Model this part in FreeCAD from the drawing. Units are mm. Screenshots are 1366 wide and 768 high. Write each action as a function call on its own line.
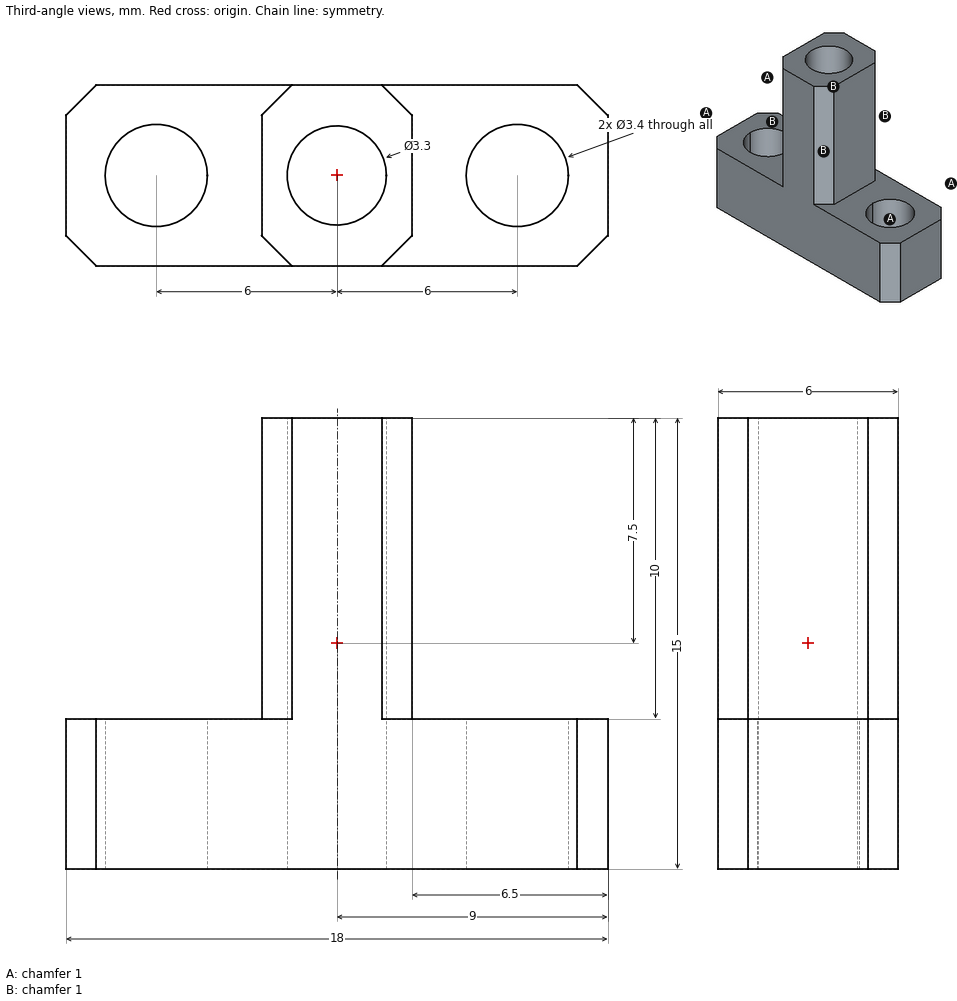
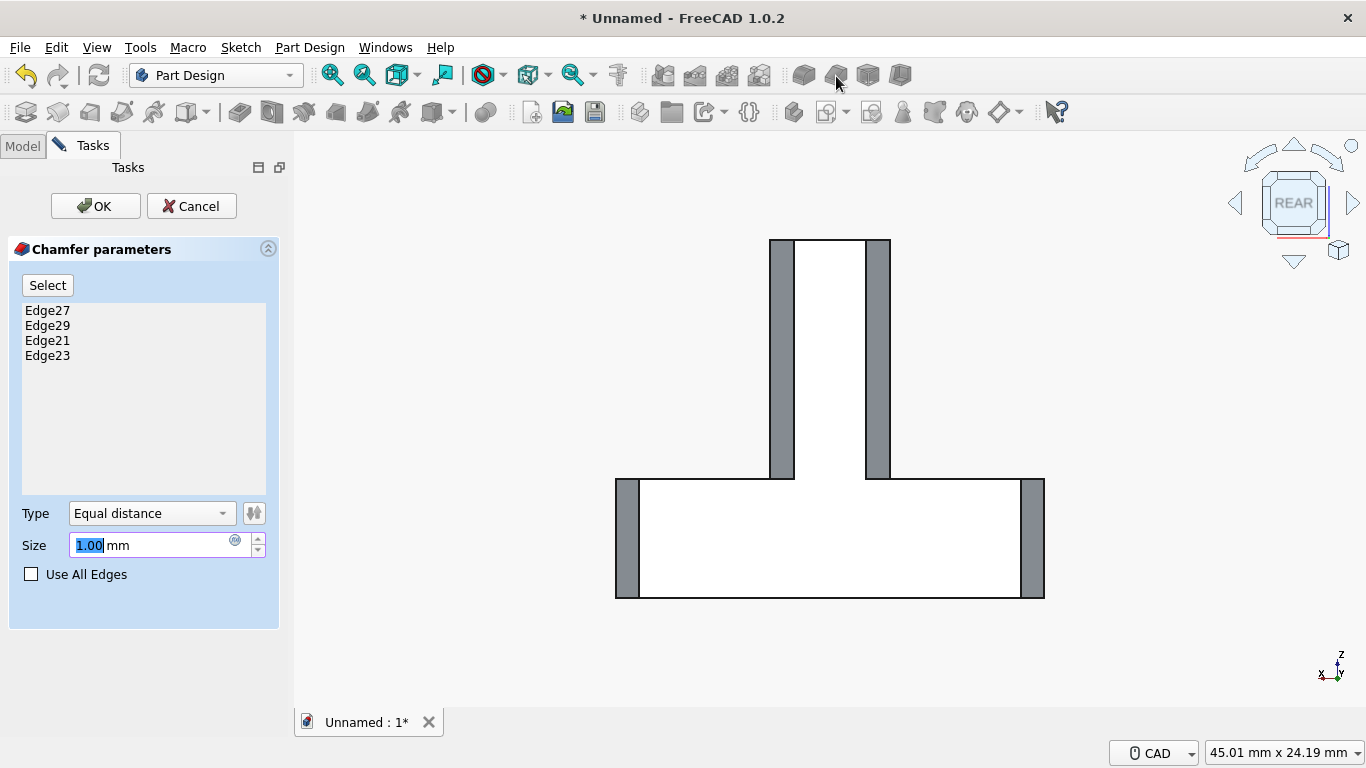
text(1)
key(Tab)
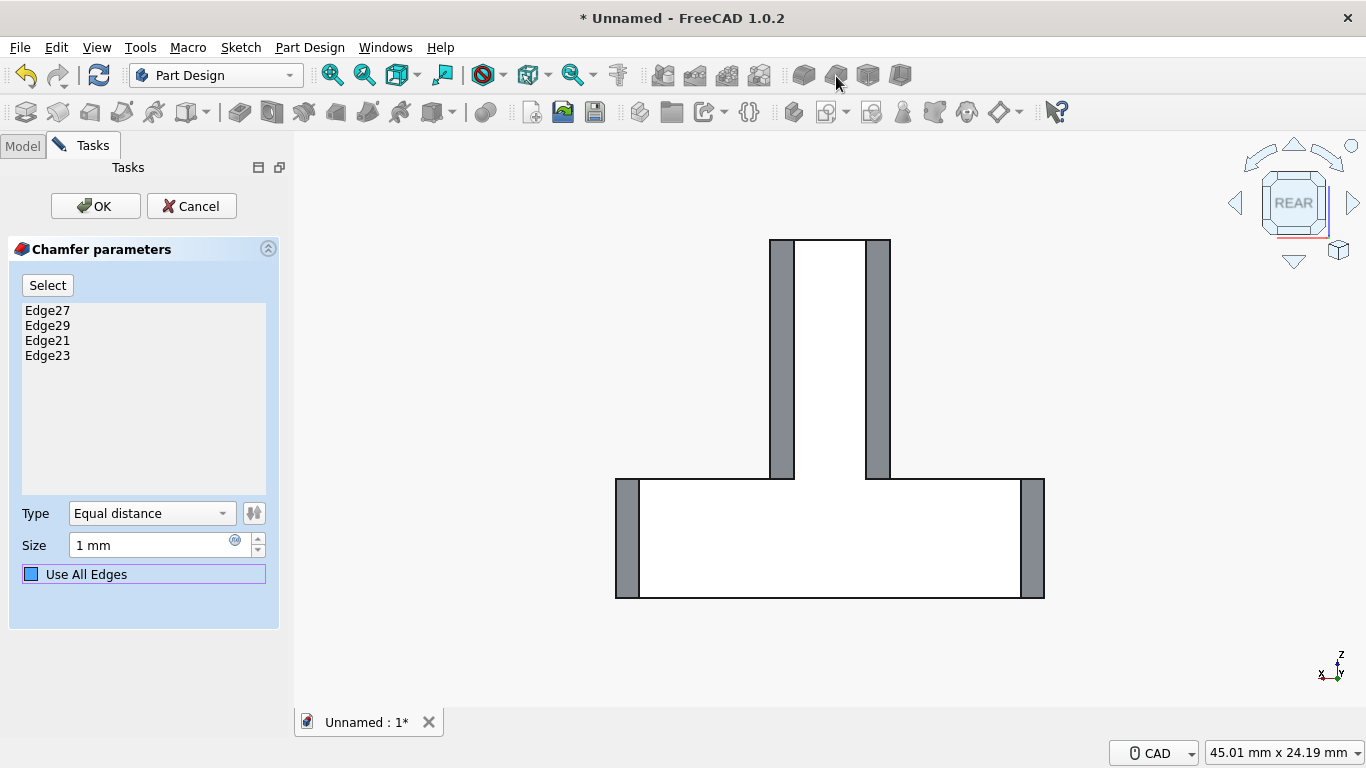
click(96, 206)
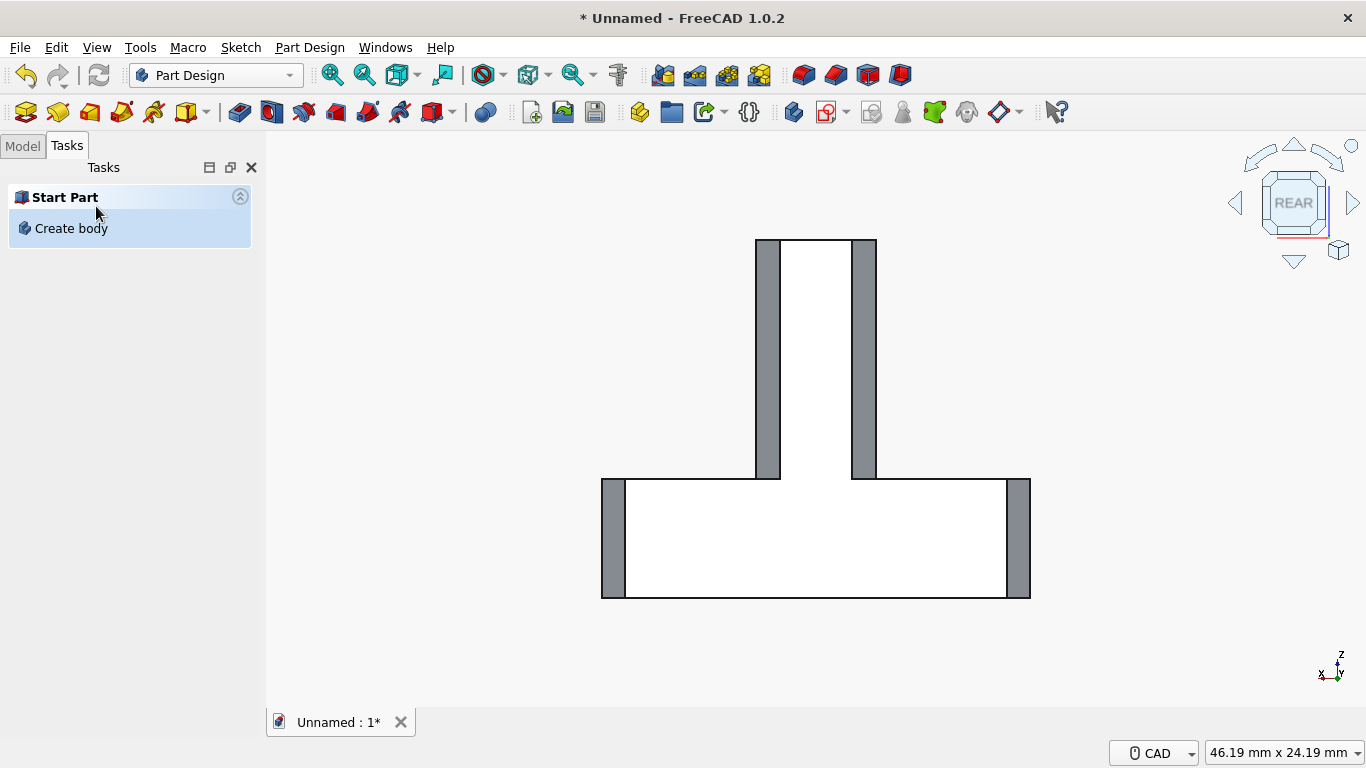
key(0)